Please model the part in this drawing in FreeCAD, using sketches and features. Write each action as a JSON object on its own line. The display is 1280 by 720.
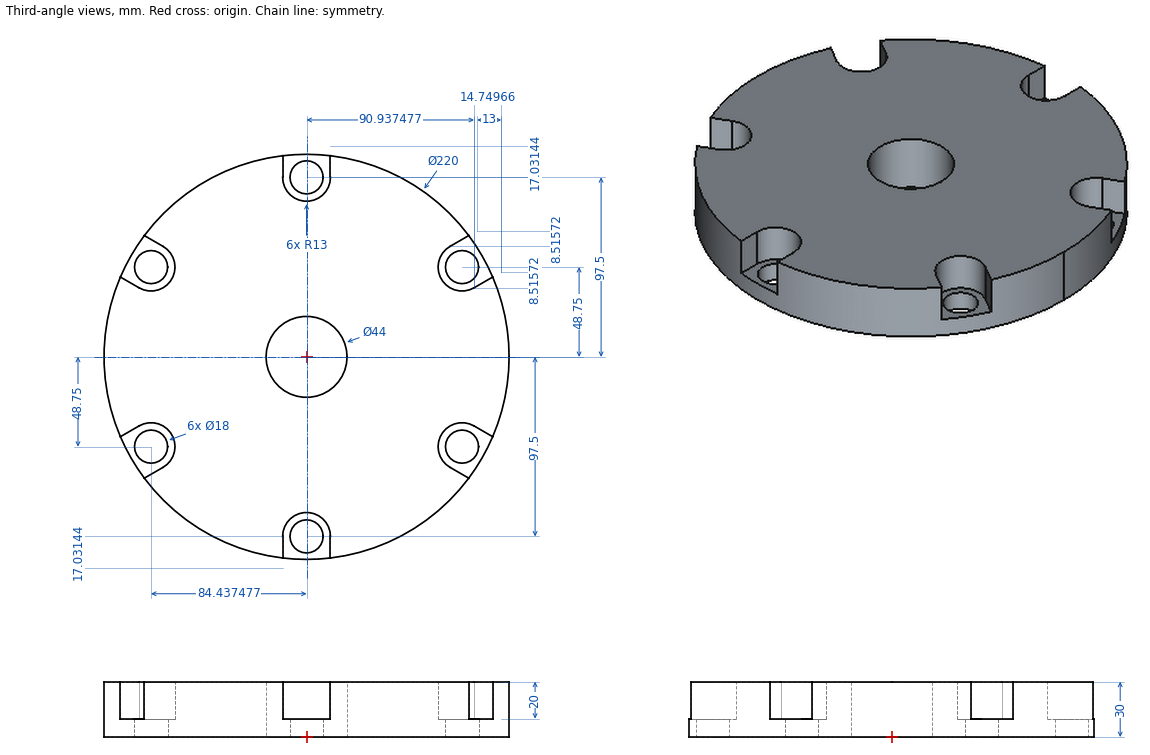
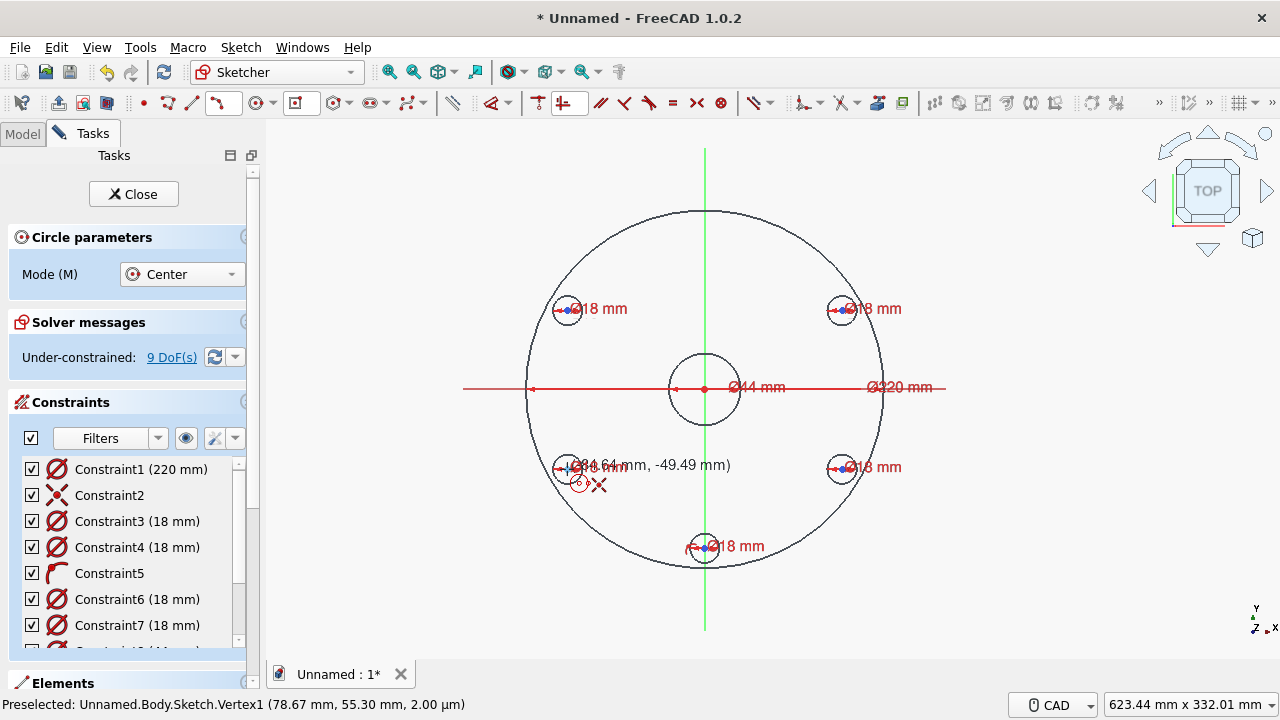
{"action": "scroll", "coordinate": [705, 231], "scroll_direction": "up", "scroll_amount": 3}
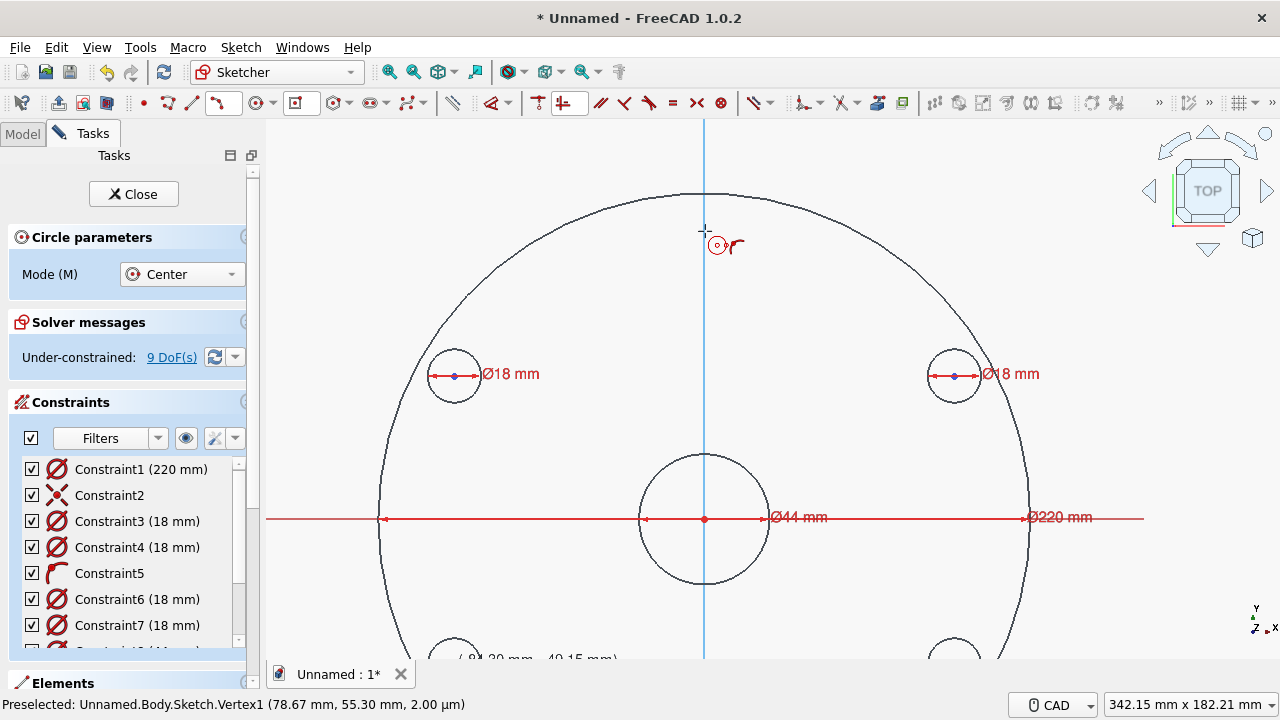
{"action": "left_click", "coordinate": [704, 230]}
{"action": "mouse_move", "coordinate": [723, 212]}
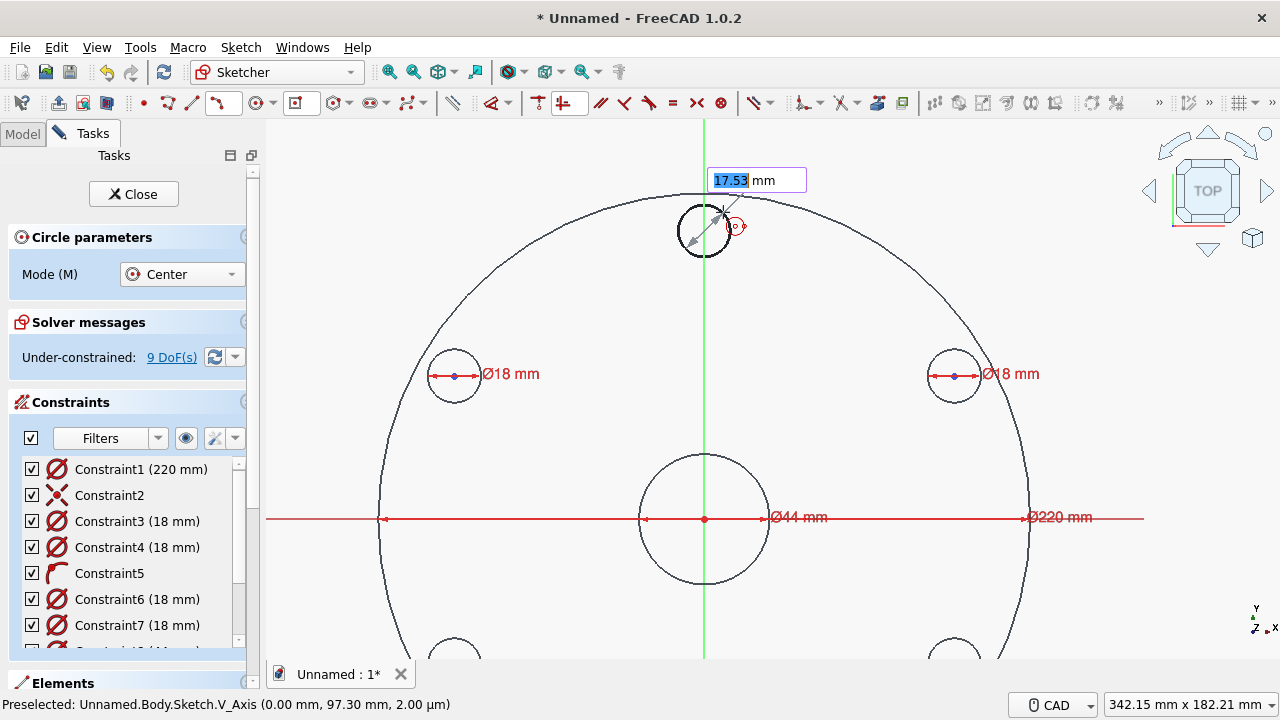
{"action": "type", "text": "18"}
{"action": "key", "text": "Return"}
{"action": "key", "text": "Escape"}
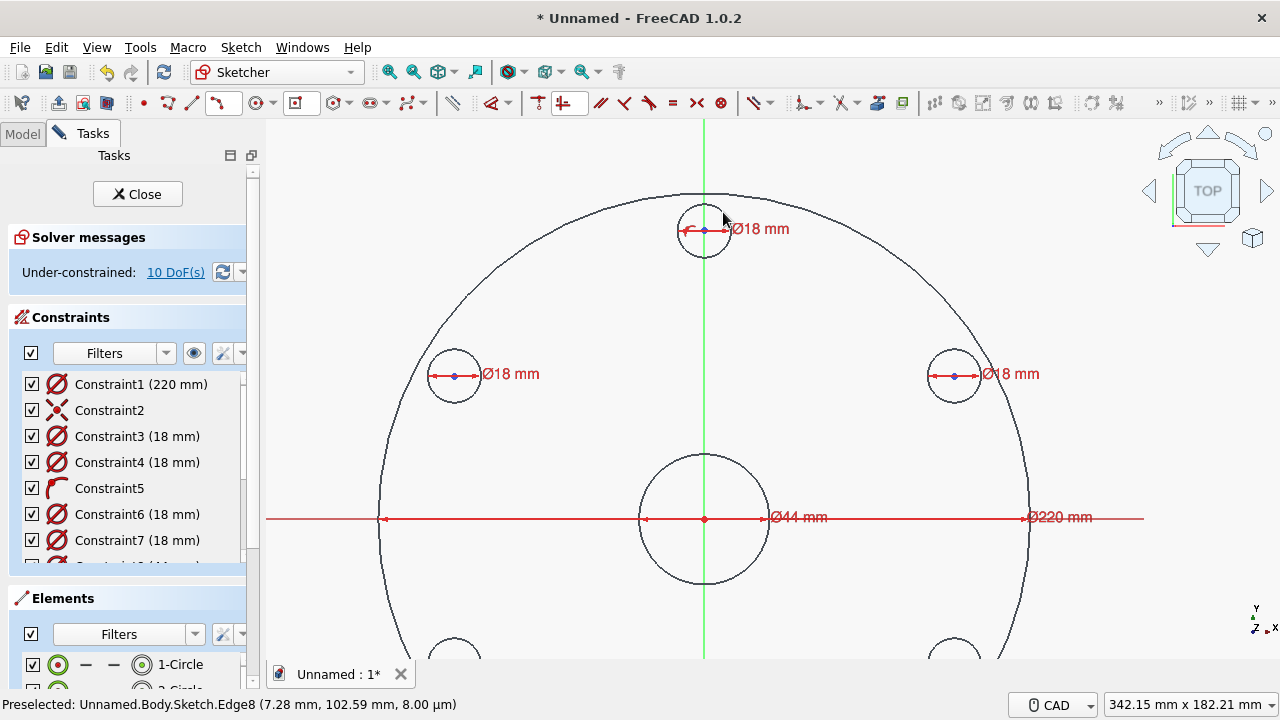
{"action": "scroll", "coordinate": [705, 230], "scroll_direction": "down", "scroll_amount": 3}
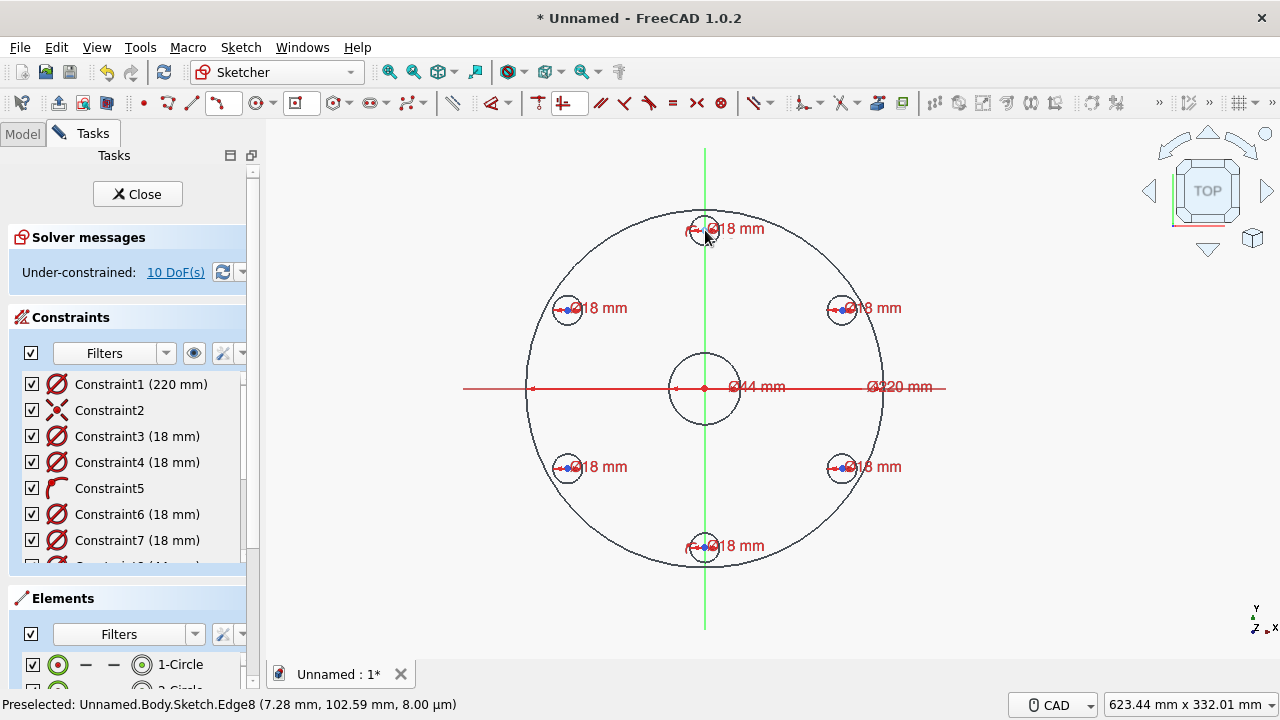
{"action": "left_click", "coordinate": [568, 469]}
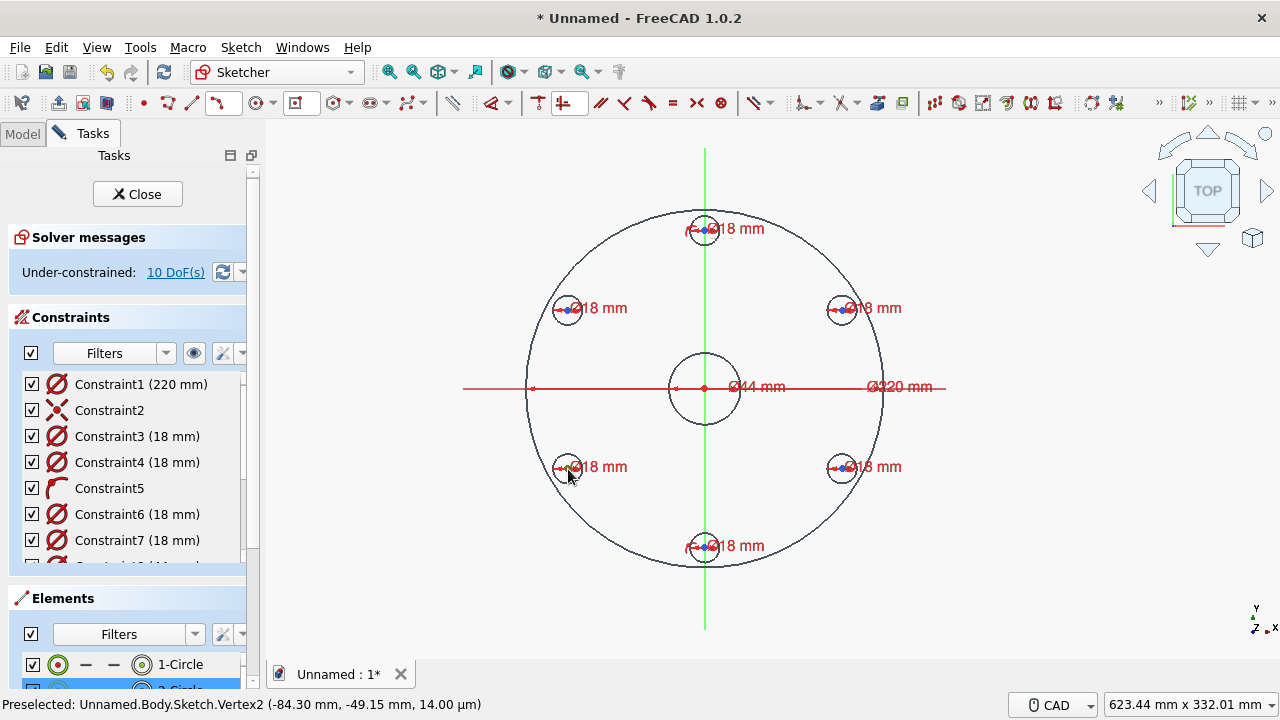
{"action": "left_click", "coordinate": [842, 469]}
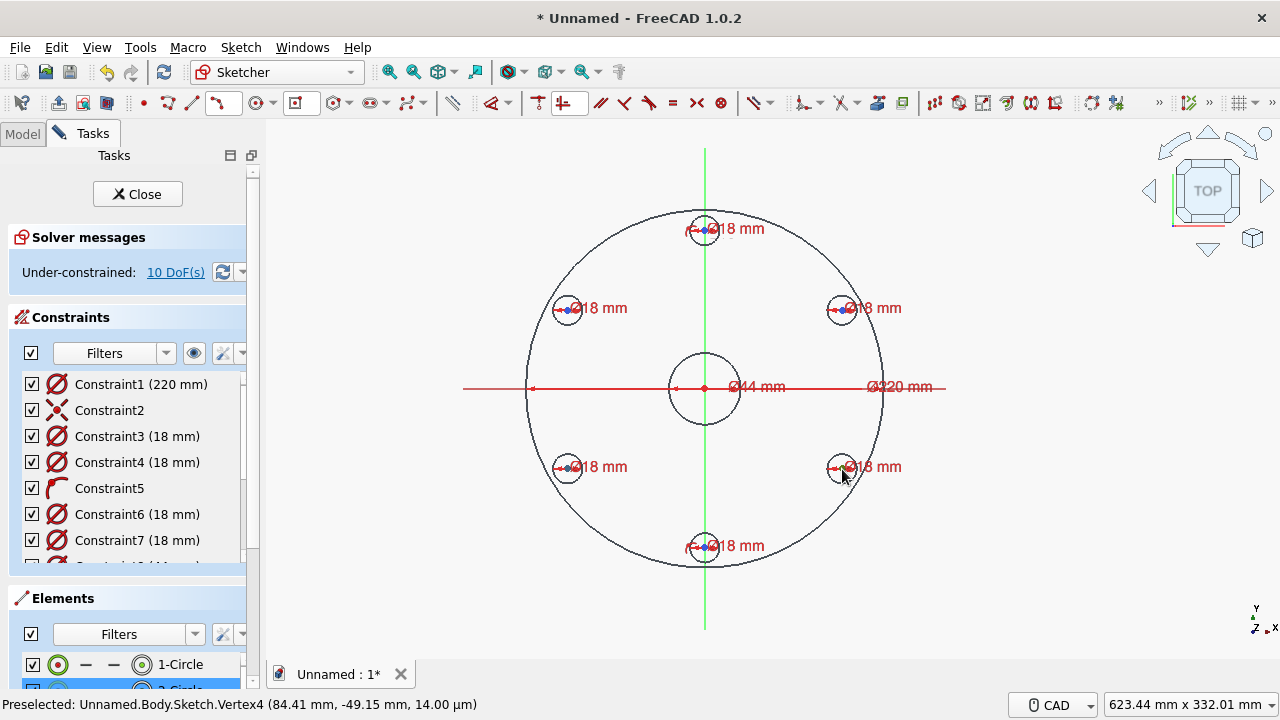
{"action": "left_click", "coordinate": [705, 493]}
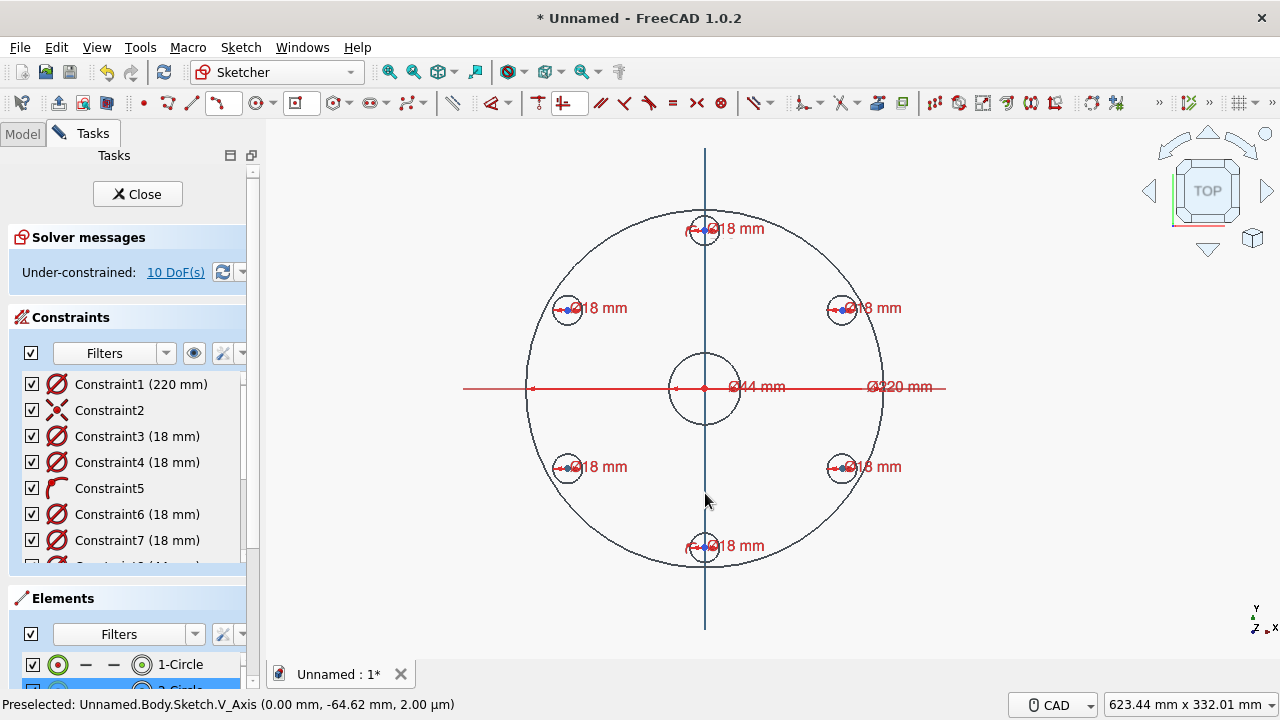
{"action": "left_click", "coordinate": [698, 104]}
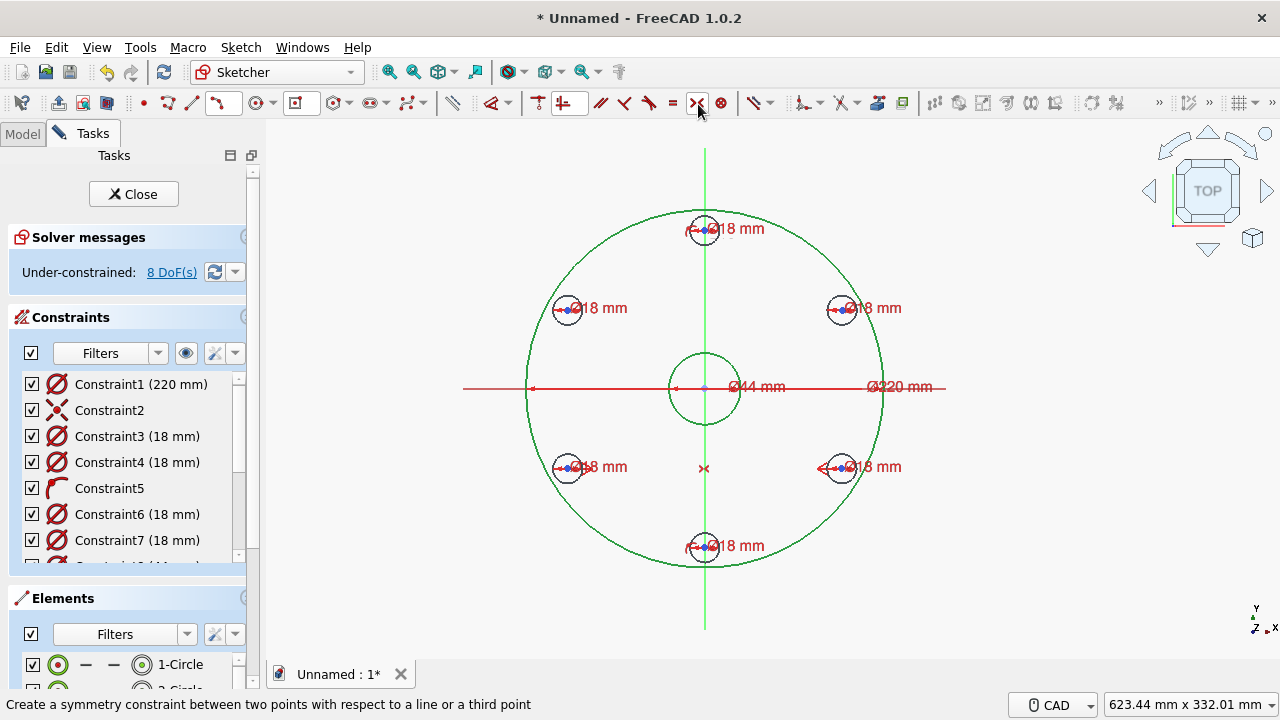
{"action": "left_click", "coordinate": [568, 469]}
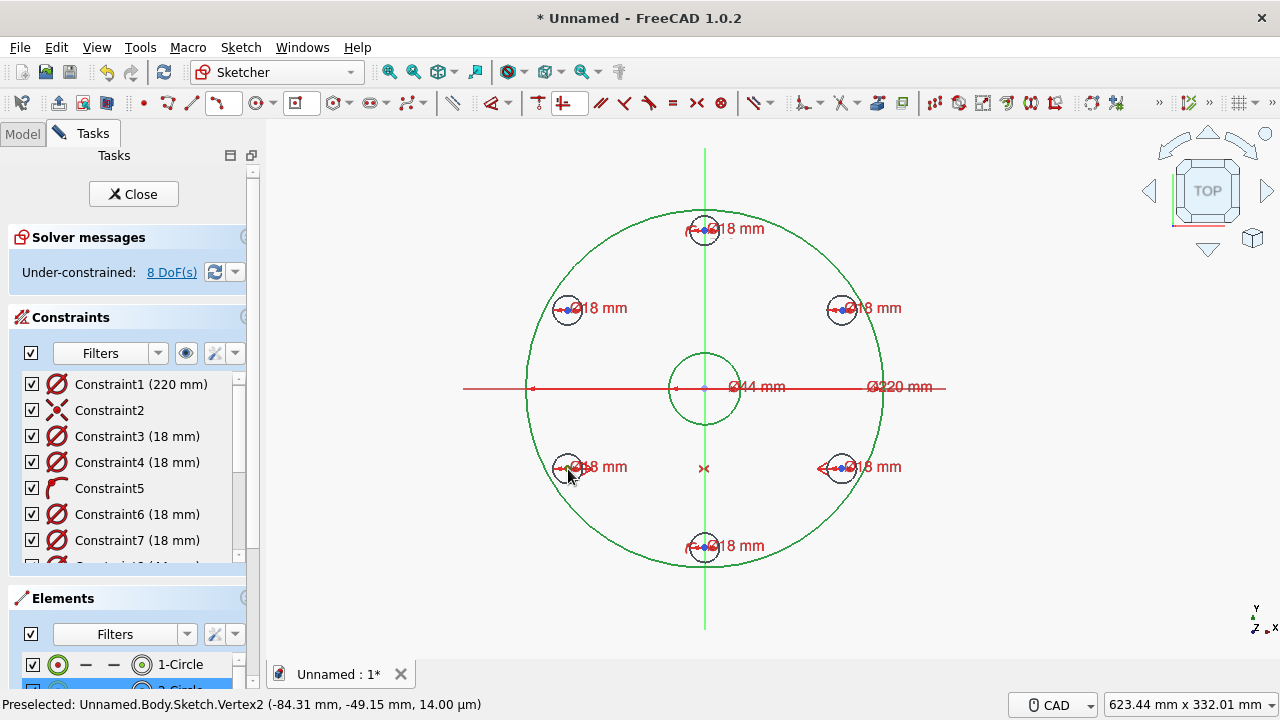
{"action": "left_click", "coordinate": [568, 310]}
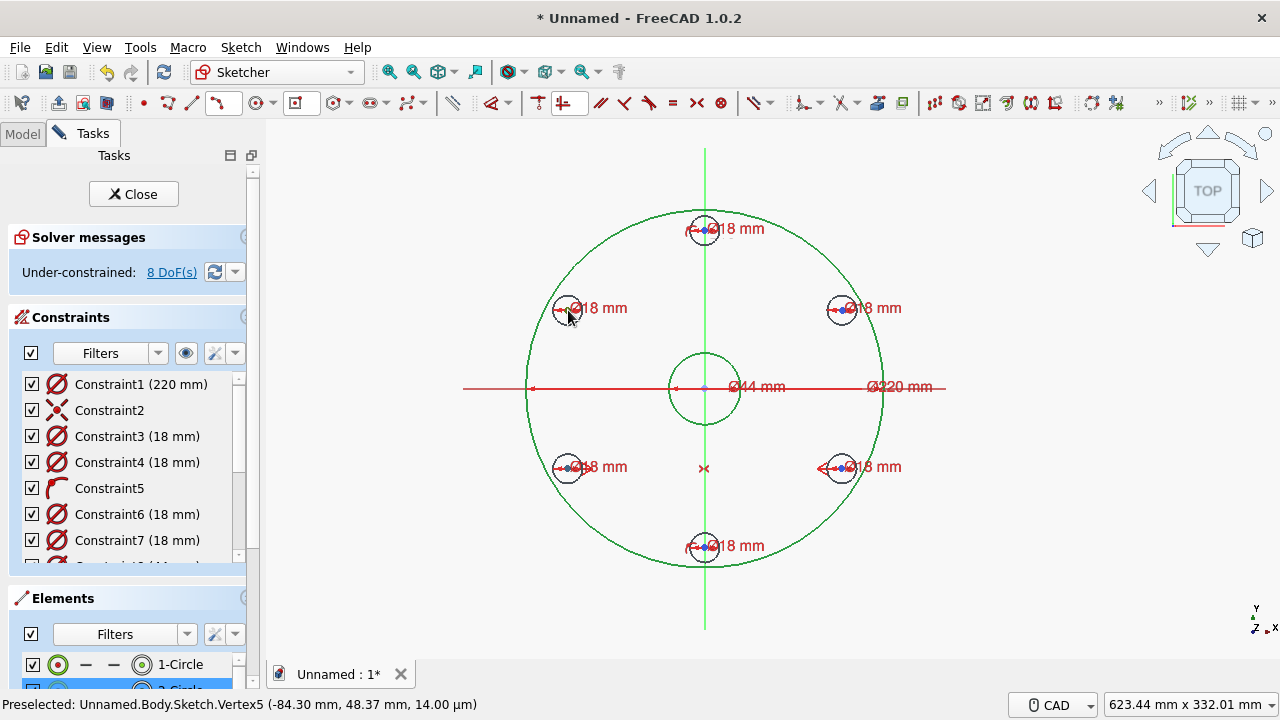
{"action": "left_click", "coordinate": [470, 389]}